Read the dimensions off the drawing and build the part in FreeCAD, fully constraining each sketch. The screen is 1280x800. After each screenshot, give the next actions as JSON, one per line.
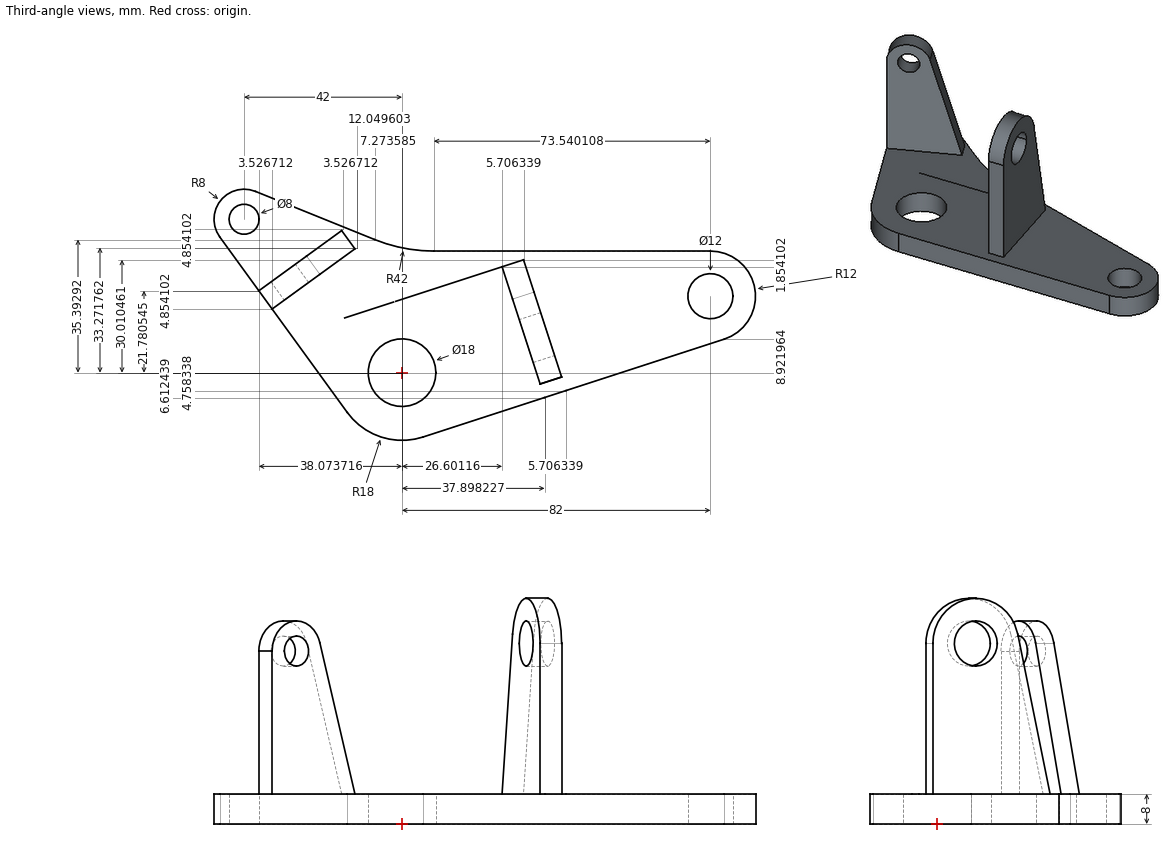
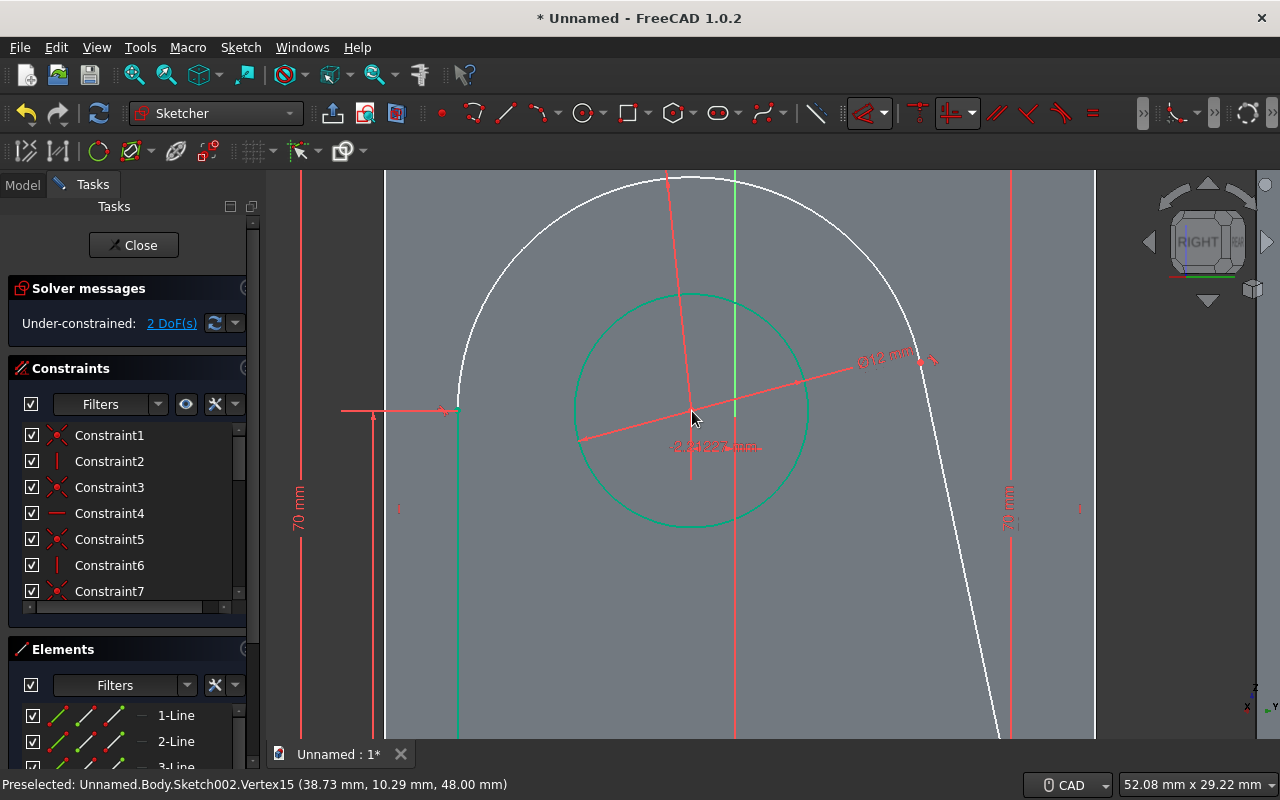
{"action": "scroll", "coordinate": [693, 411], "scroll_direction": "down", "scroll_amount": 7}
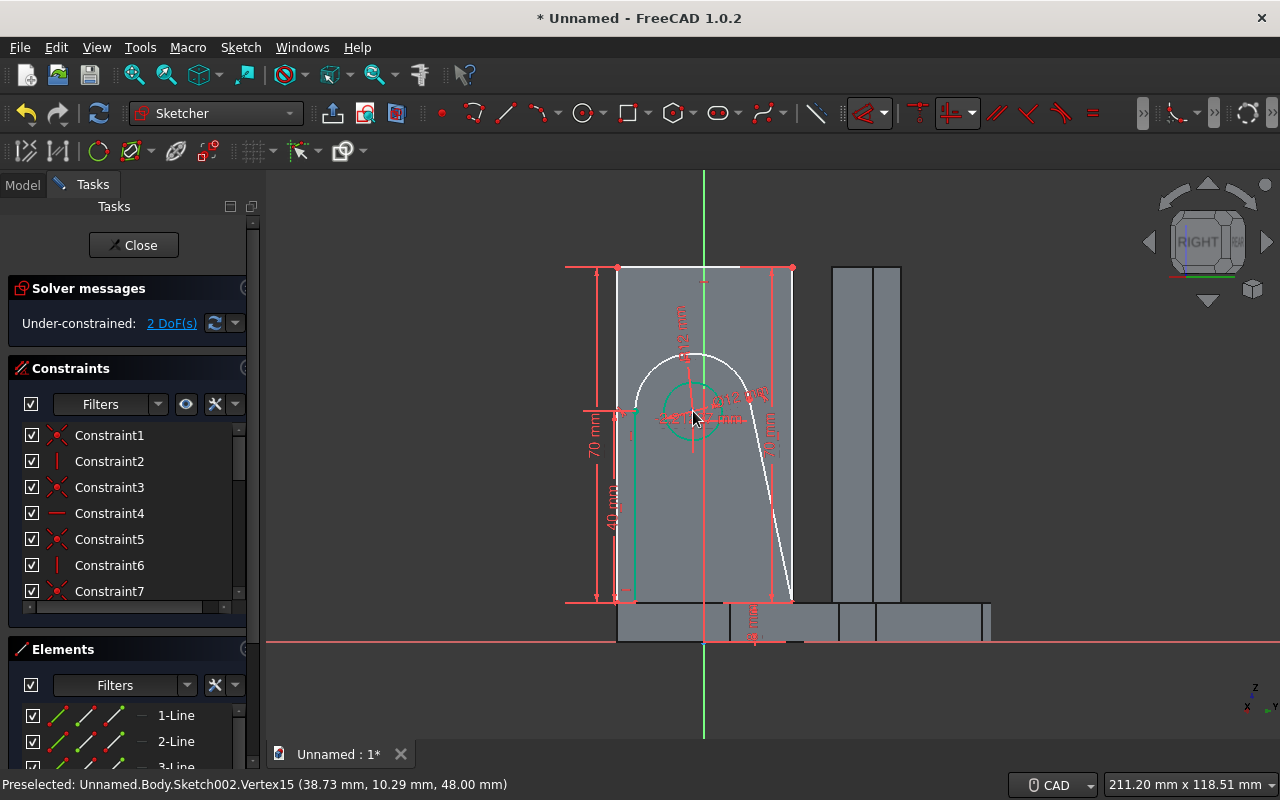
{"action": "scroll", "coordinate": [623, 603], "scroll_direction": "up", "scroll_amount": 5}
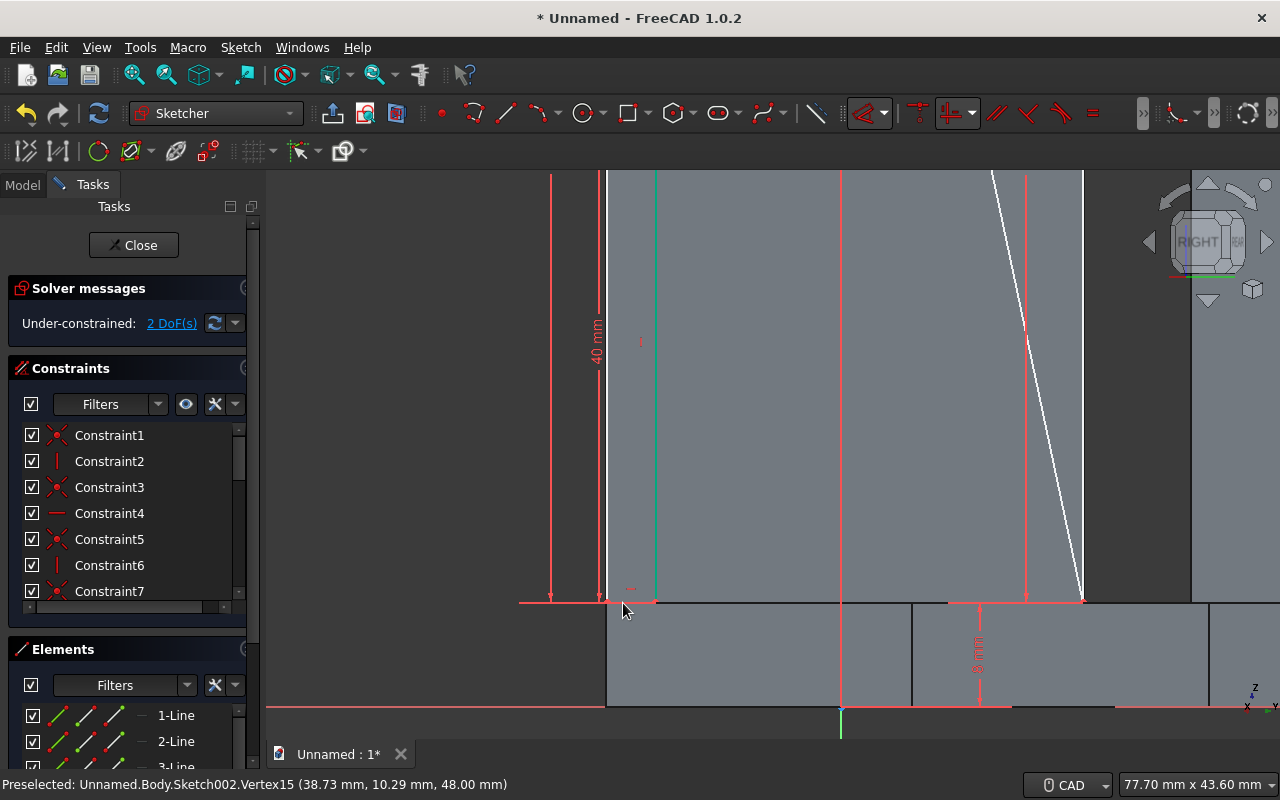
{"action": "left_click", "coordinate": [622, 603]}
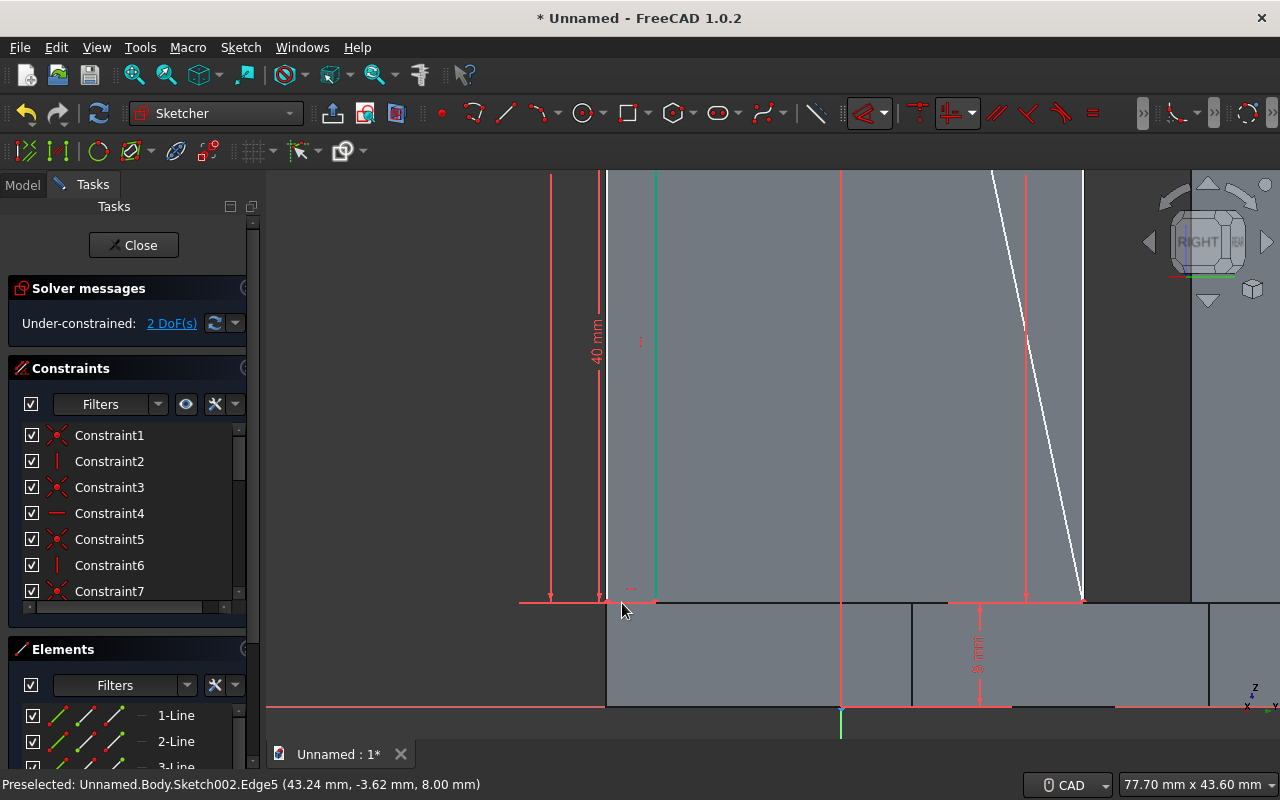
{"action": "key", "text": "l"}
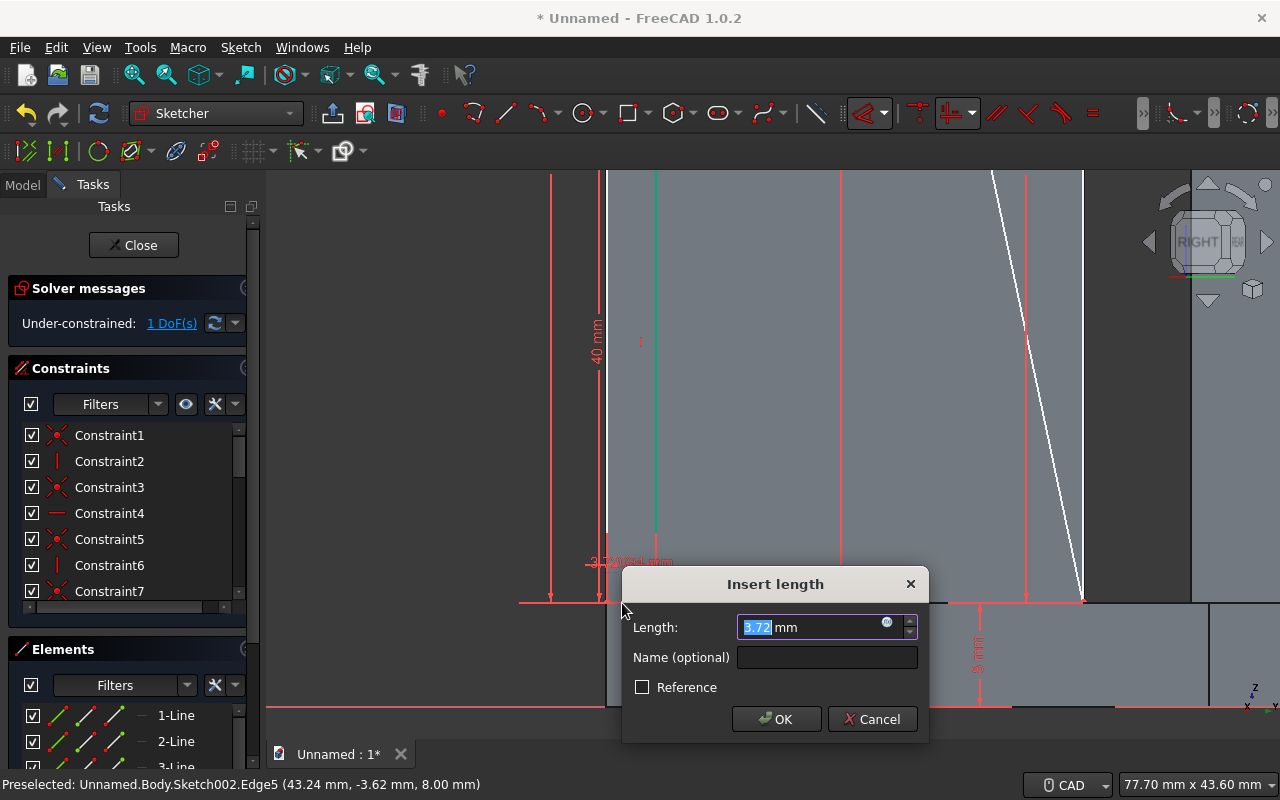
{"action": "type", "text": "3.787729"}
{"action": "key", "text": "Return"}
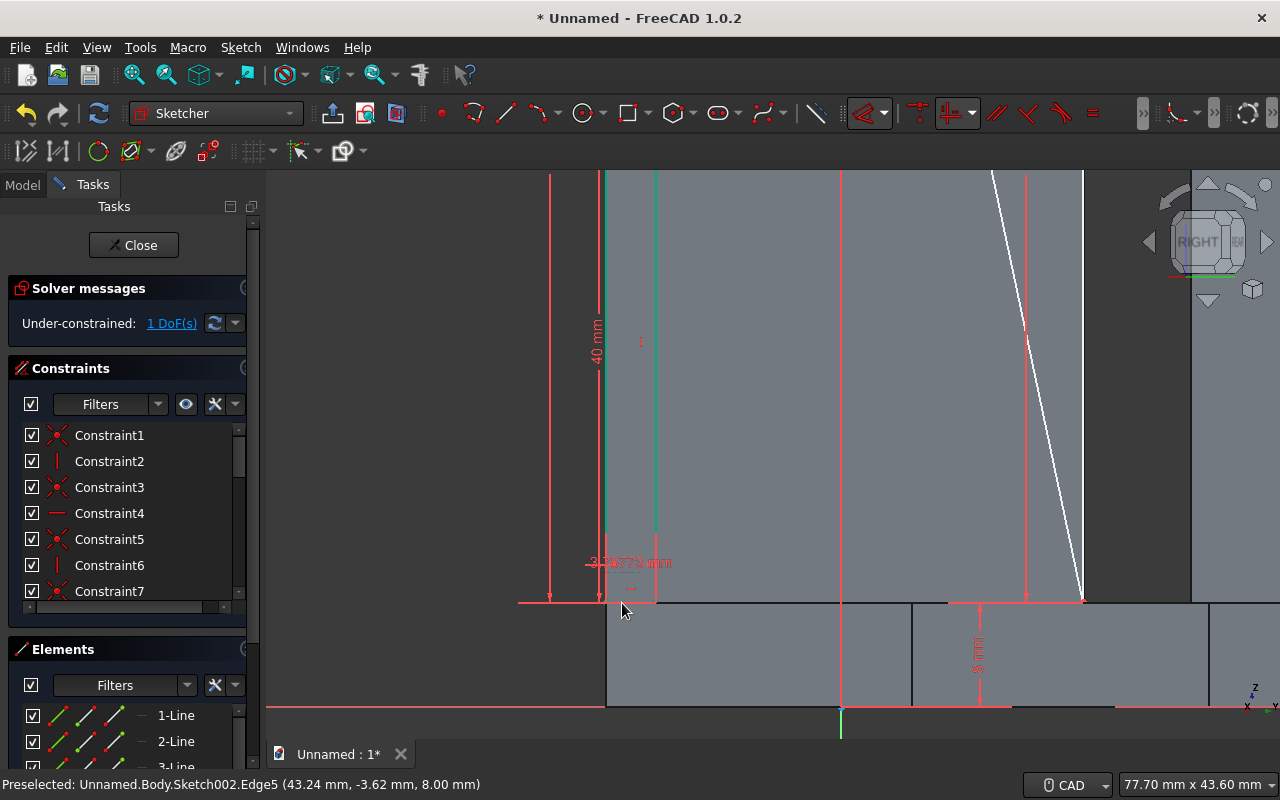
{"action": "scroll", "coordinate": [623, 604], "scroll_direction": "down", "scroll_amount": 5}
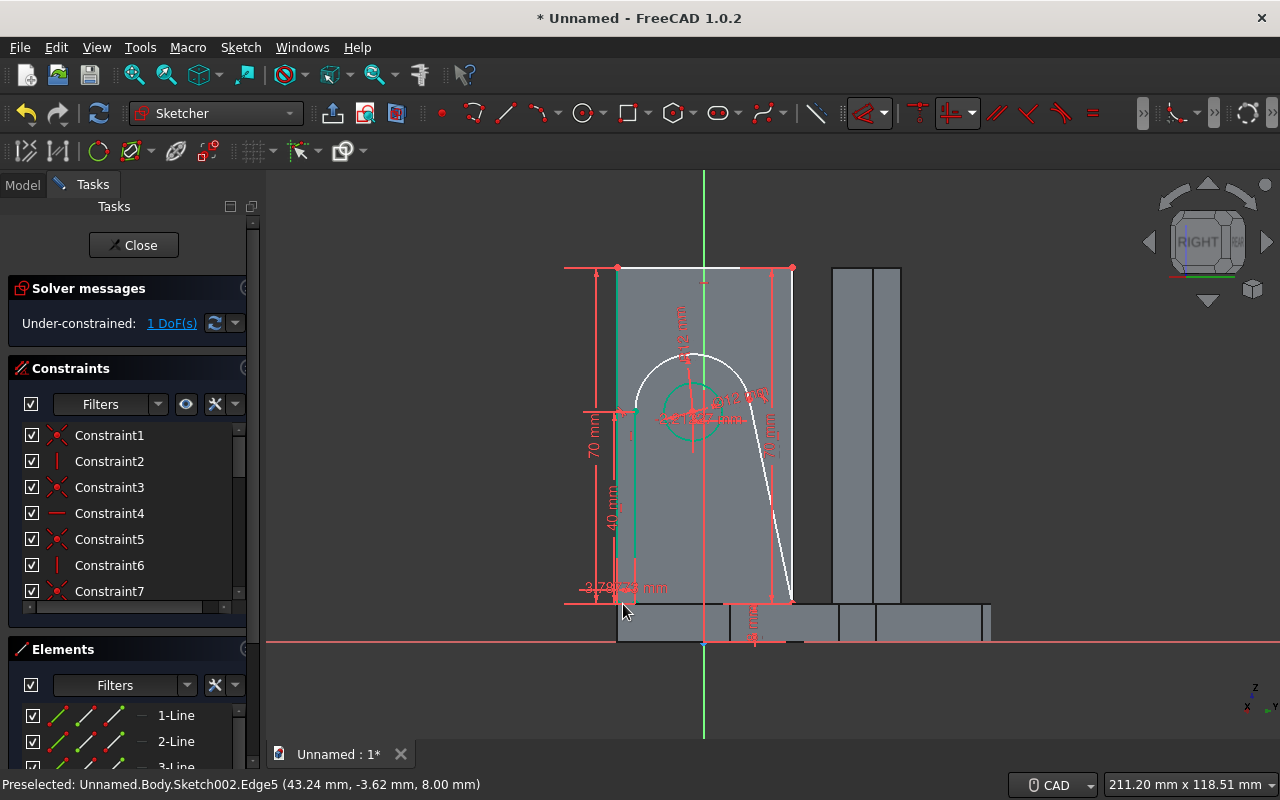
{"action": "left_click", "coordinate": [740, 268]}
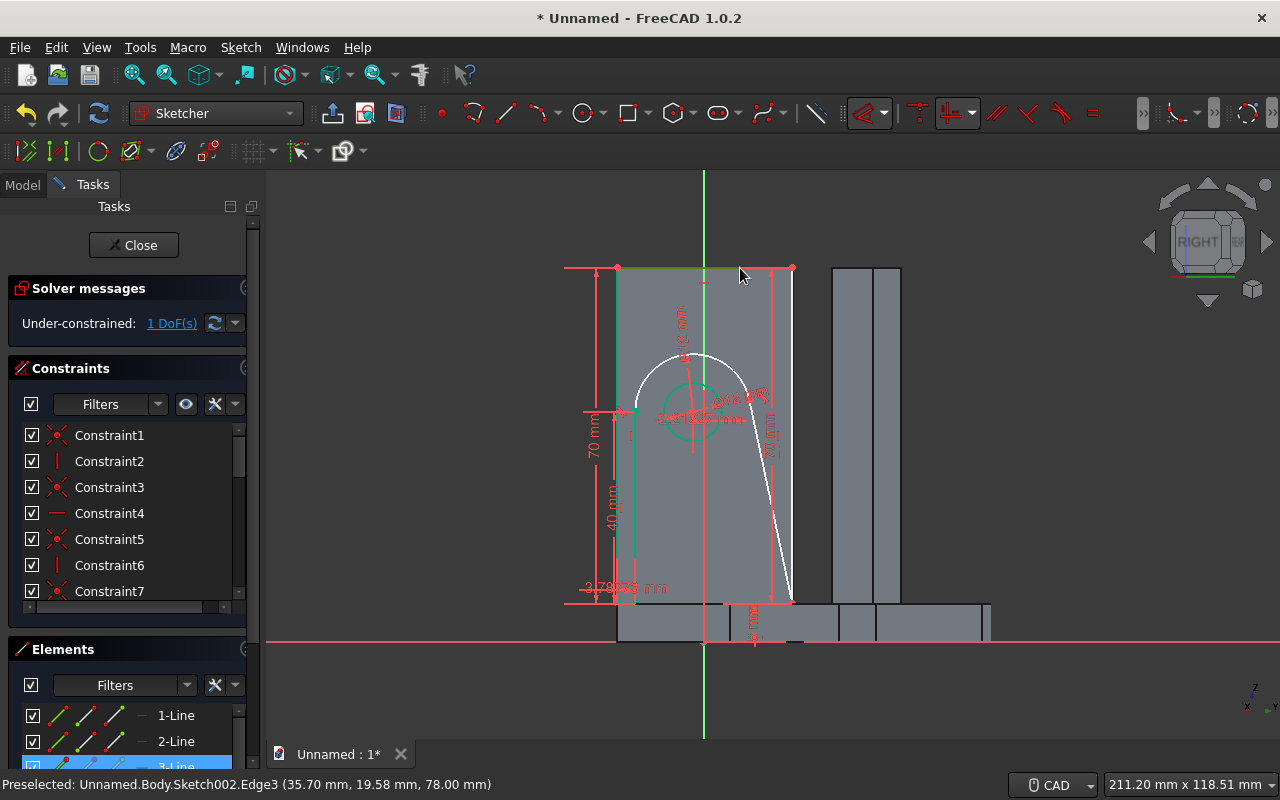
{"action": "key", "text": "l"}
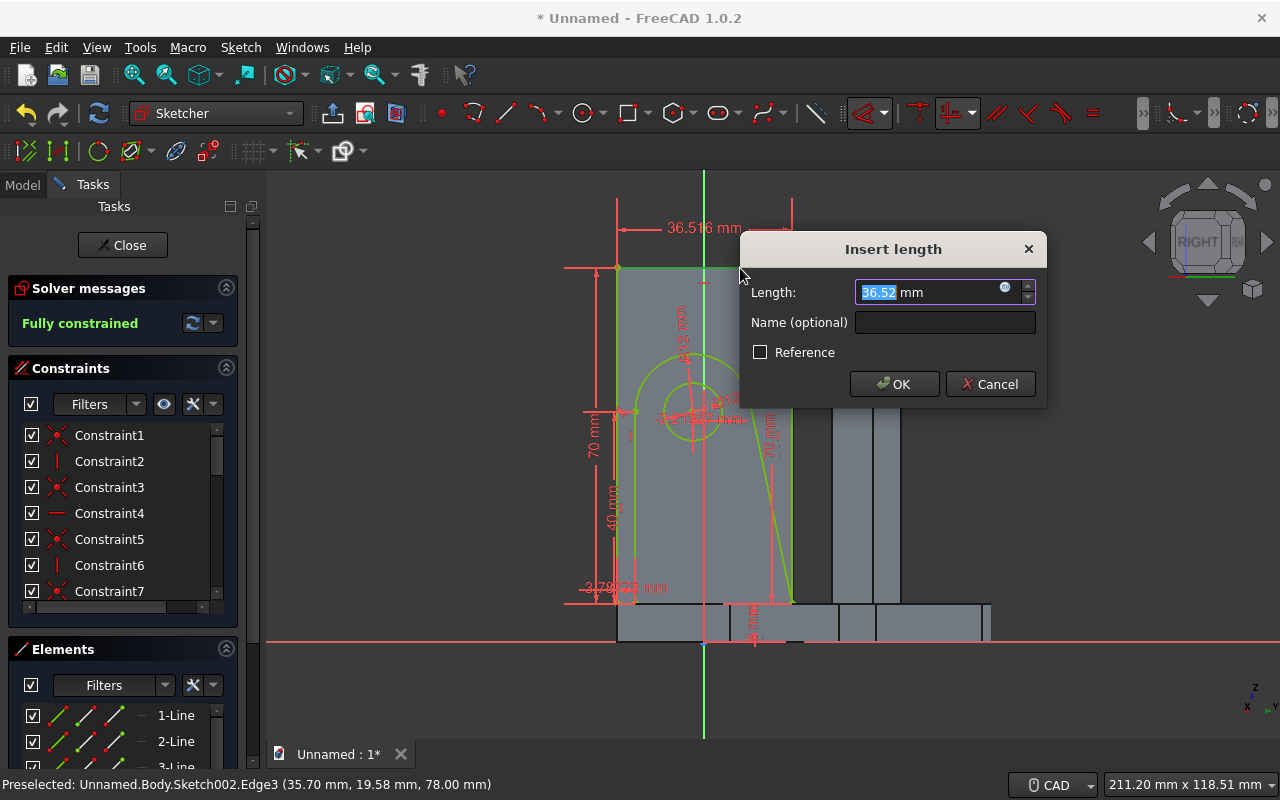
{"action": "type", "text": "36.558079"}
{"action": "key", "text": "Return"}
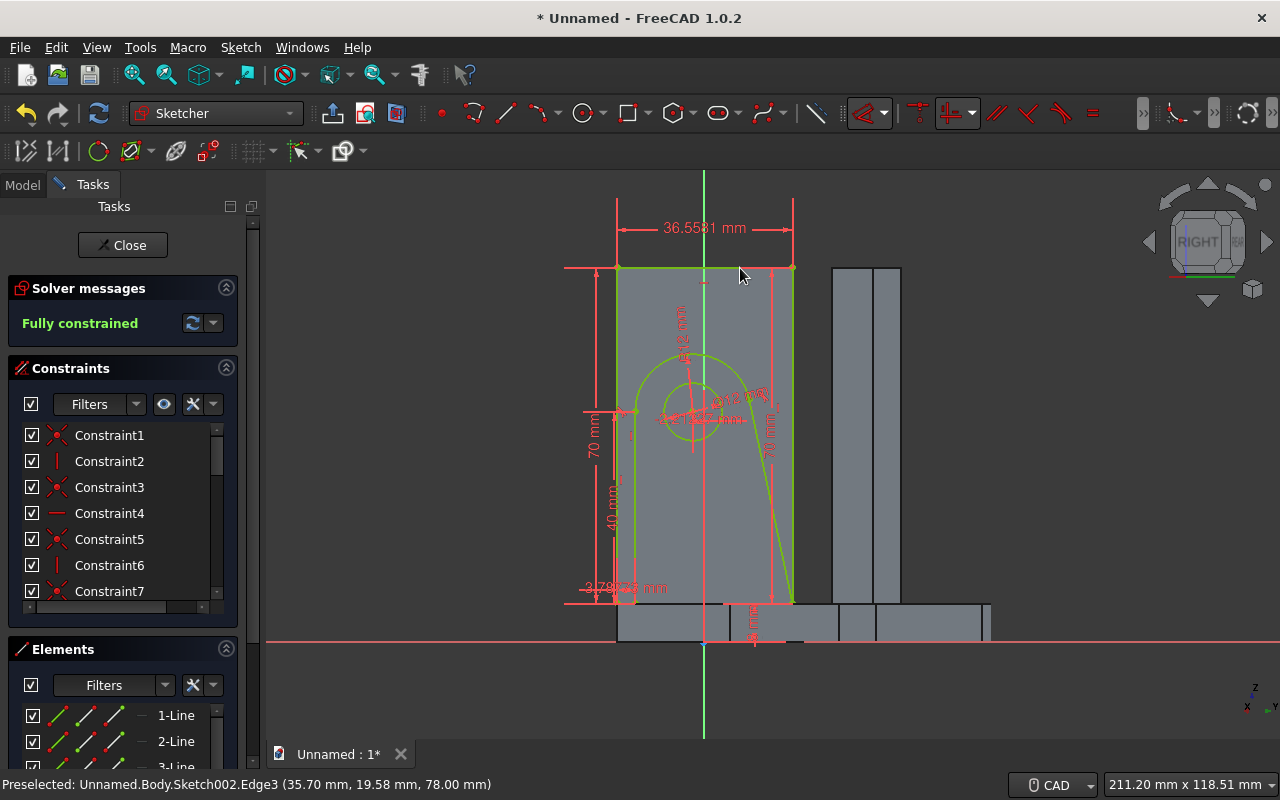
{"action": "left_click", "coordinate": [123, 245]}